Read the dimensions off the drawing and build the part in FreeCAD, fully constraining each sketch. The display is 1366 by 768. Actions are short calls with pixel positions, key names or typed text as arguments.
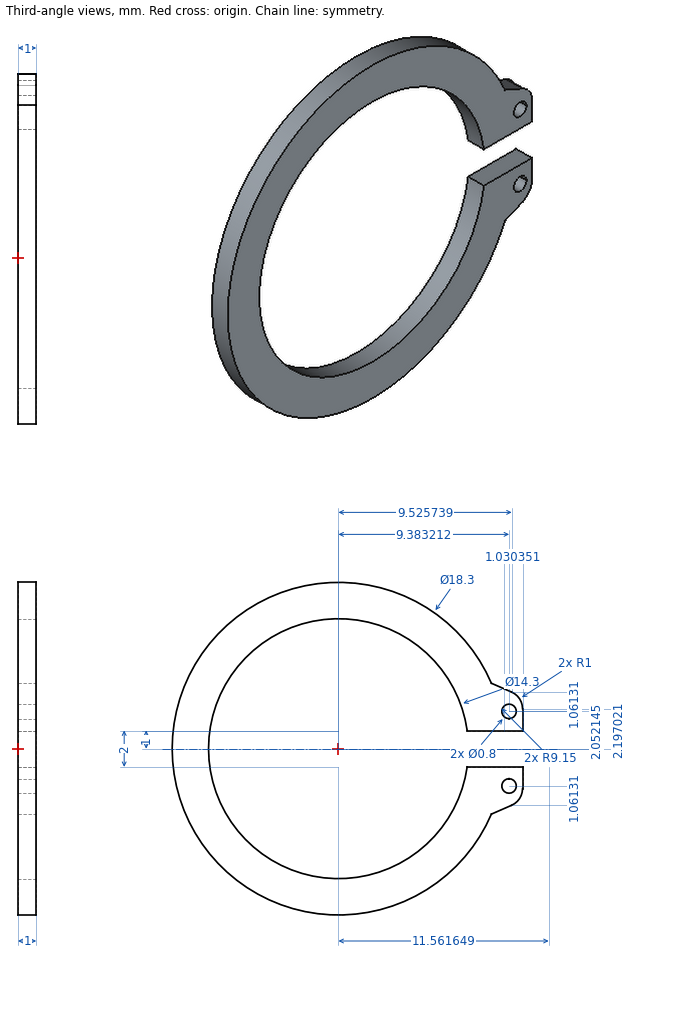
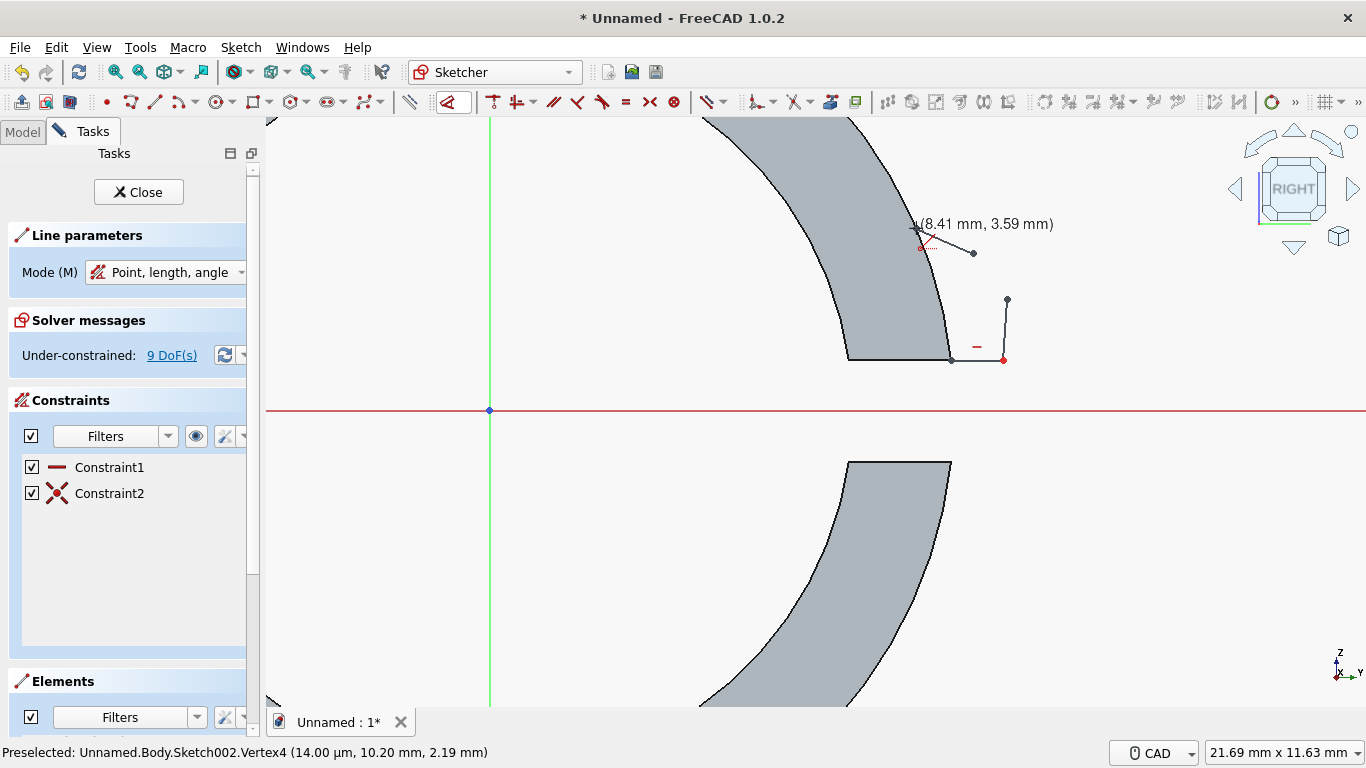
key(g)
key(3)
key(a)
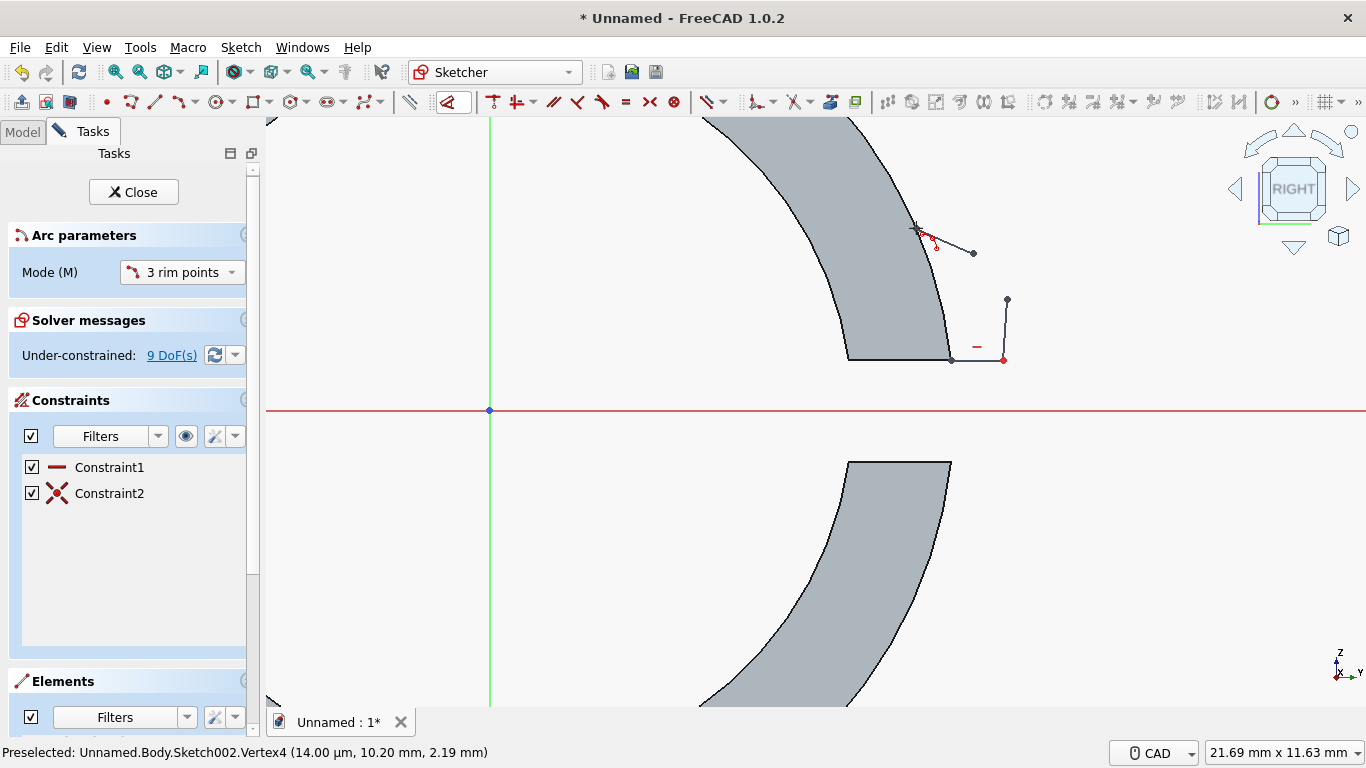
click(1007, 300)
click(973, 254)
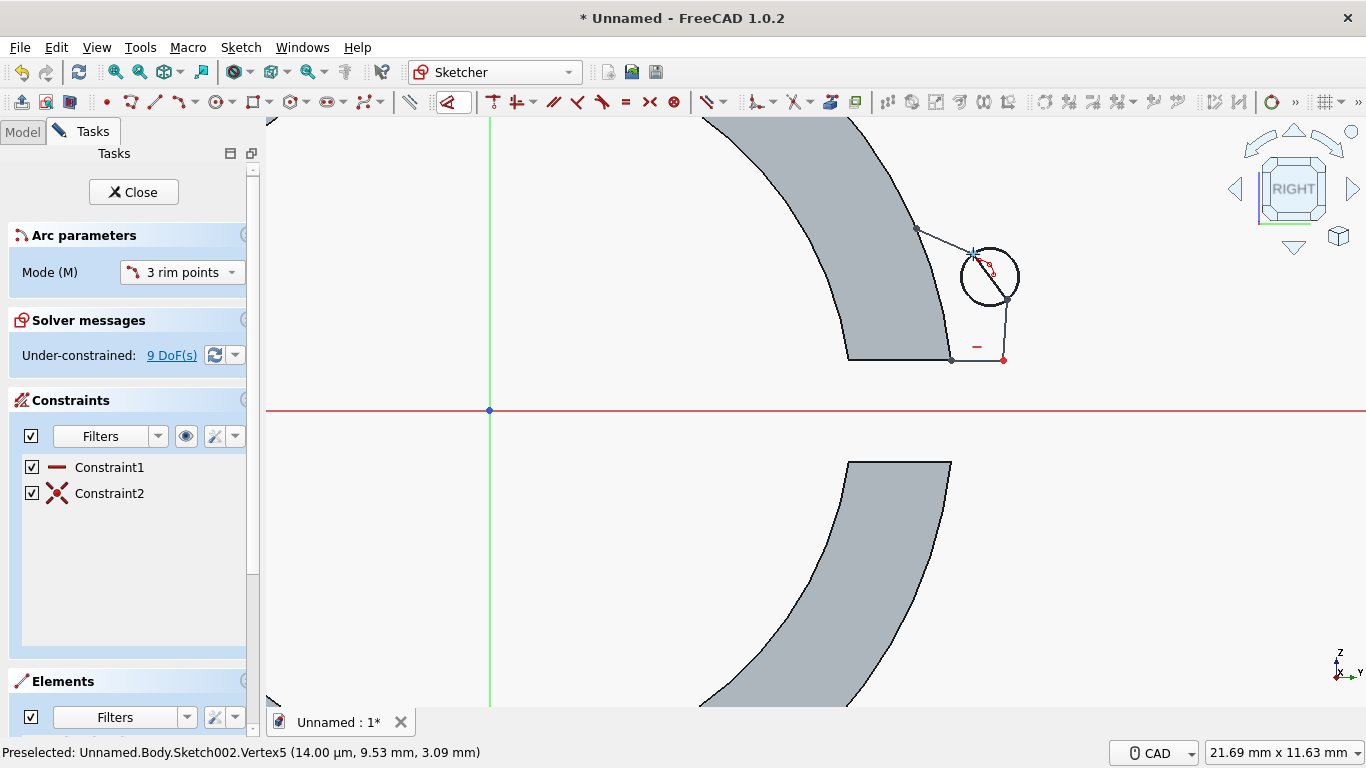
scroll(995, 272, up, 4)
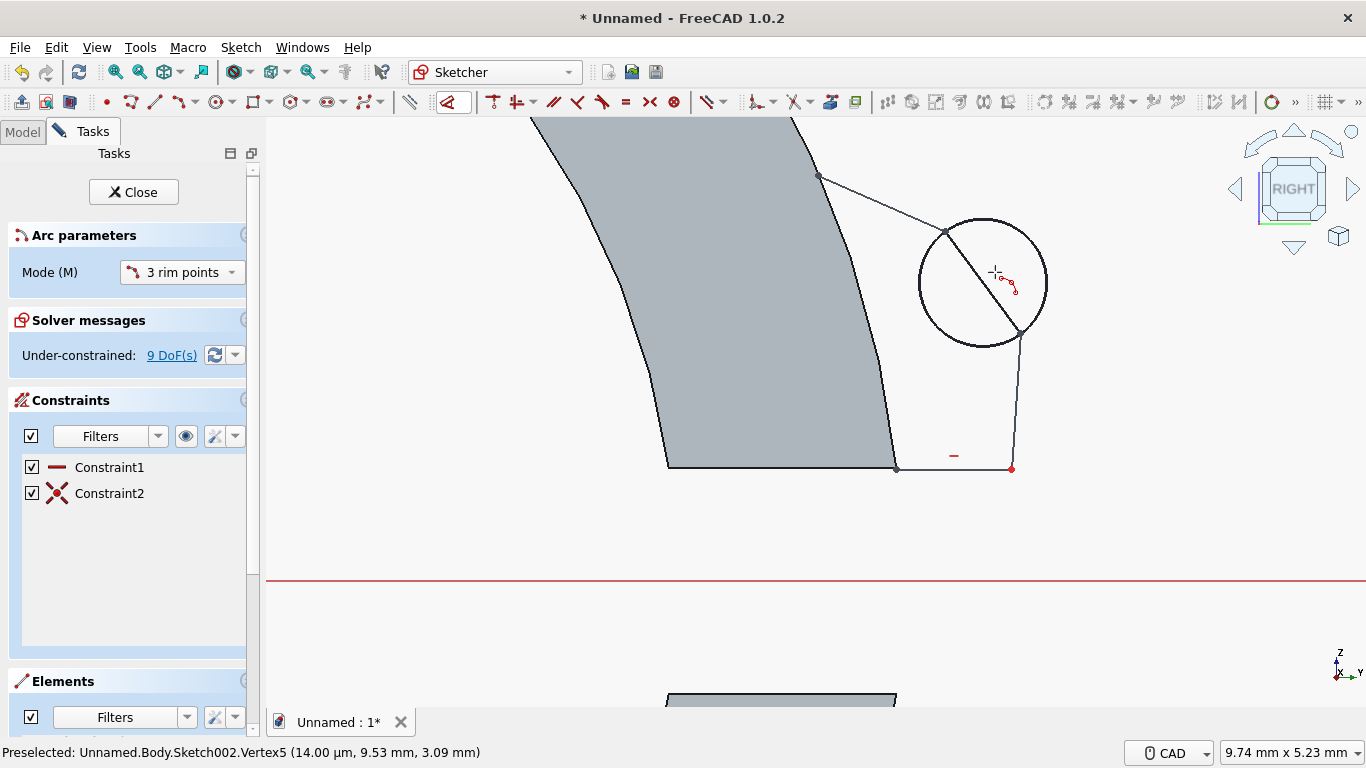
click(994, 271)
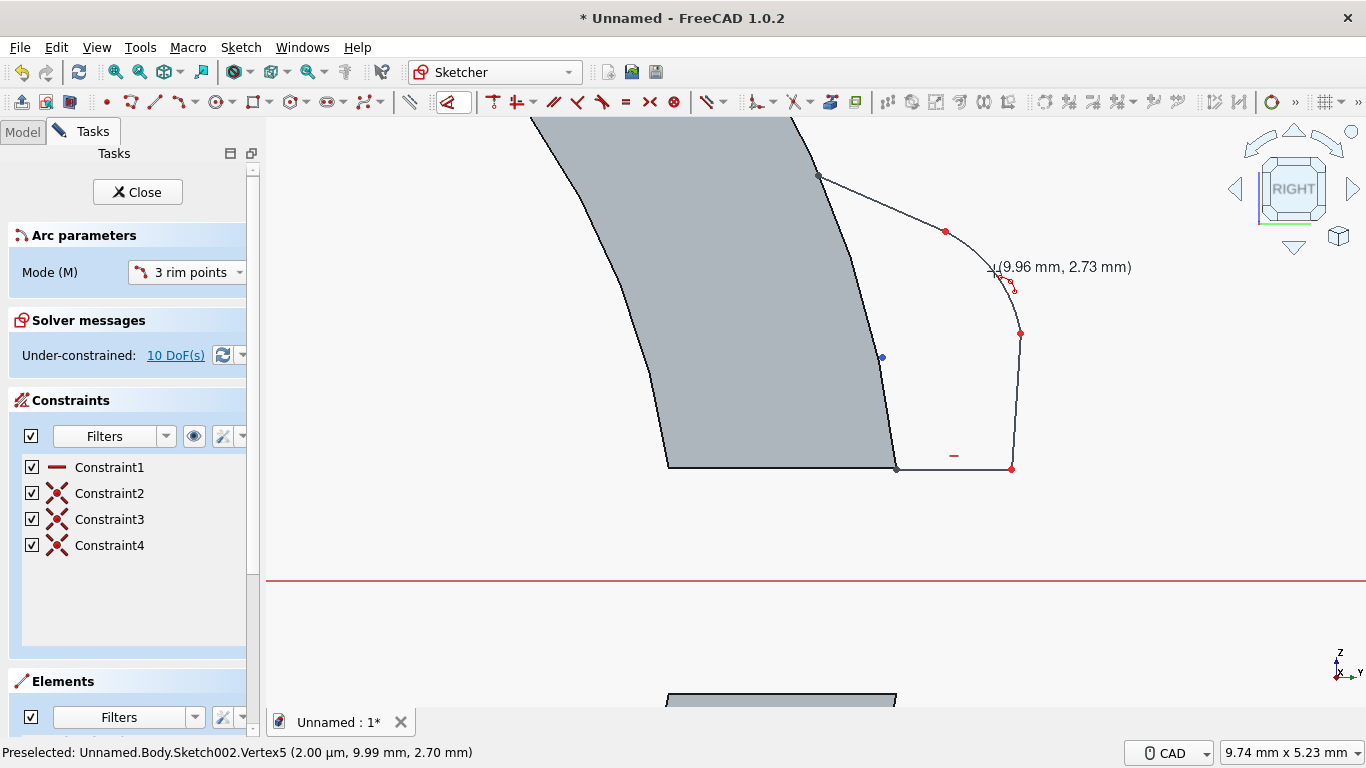
click(818, 176)
click(896, 470)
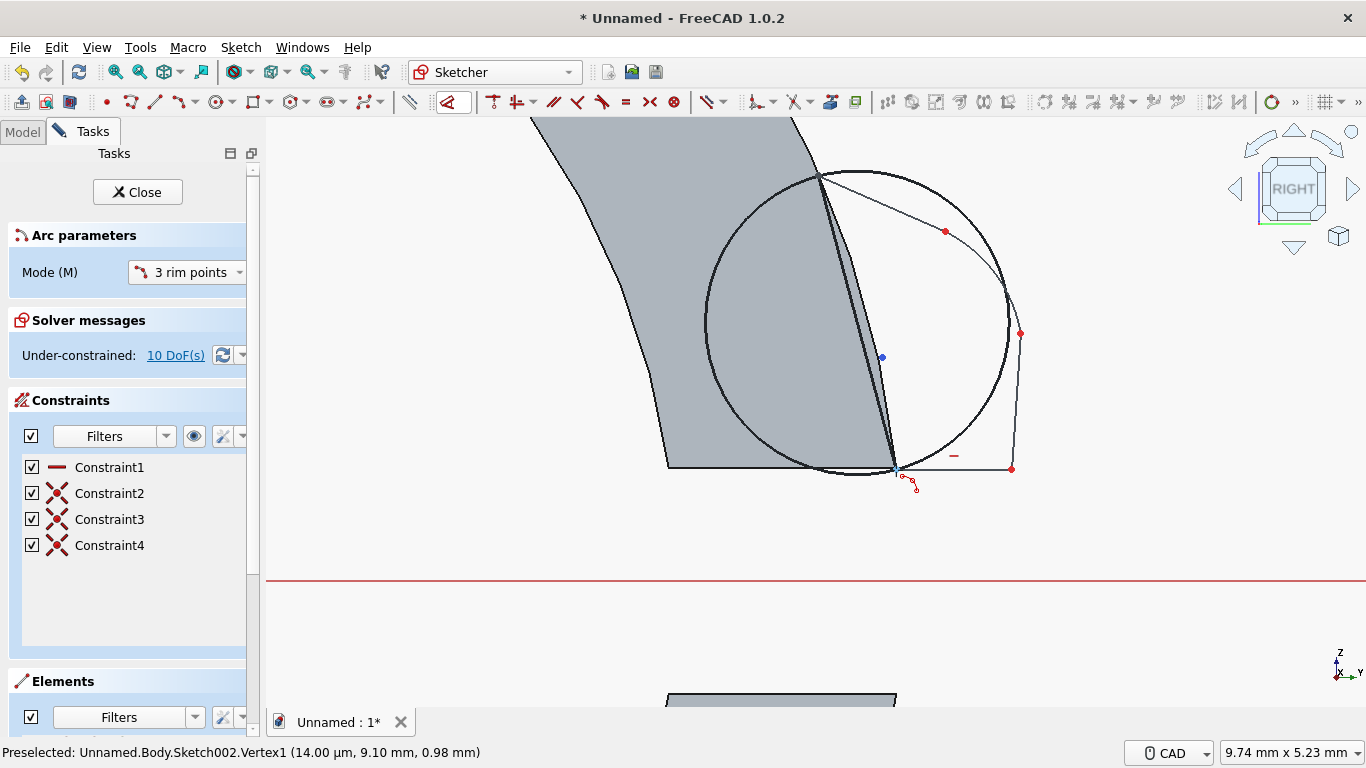
scroll(869, 318, up, 2)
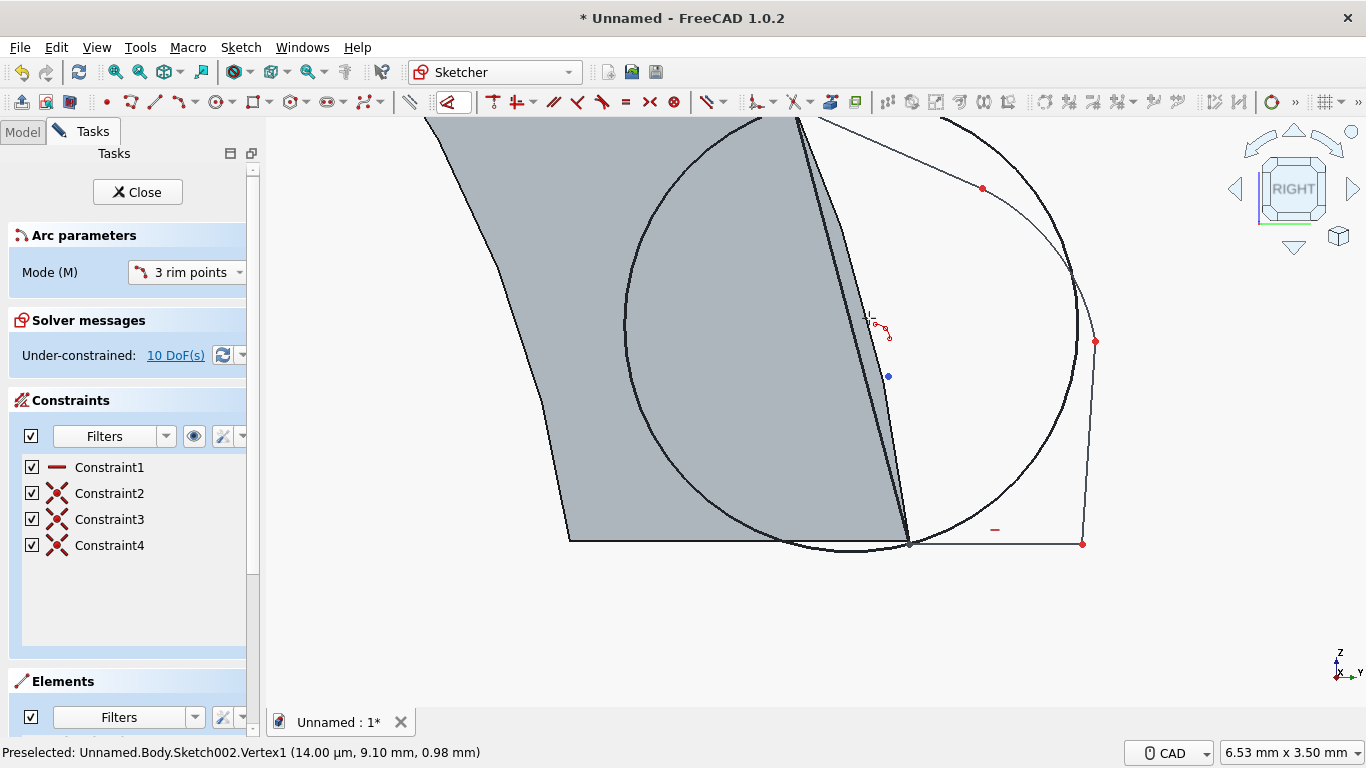
click(868, 318)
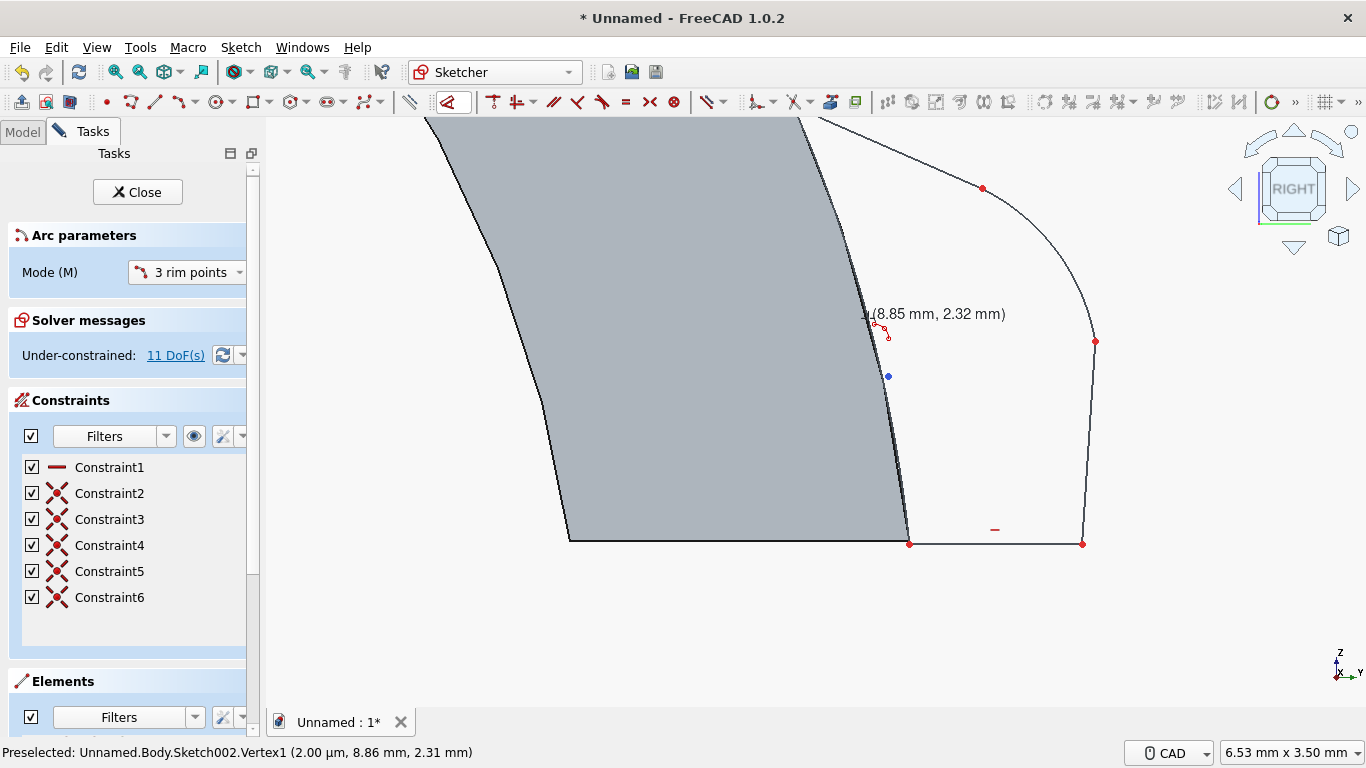
key(g)
key(l)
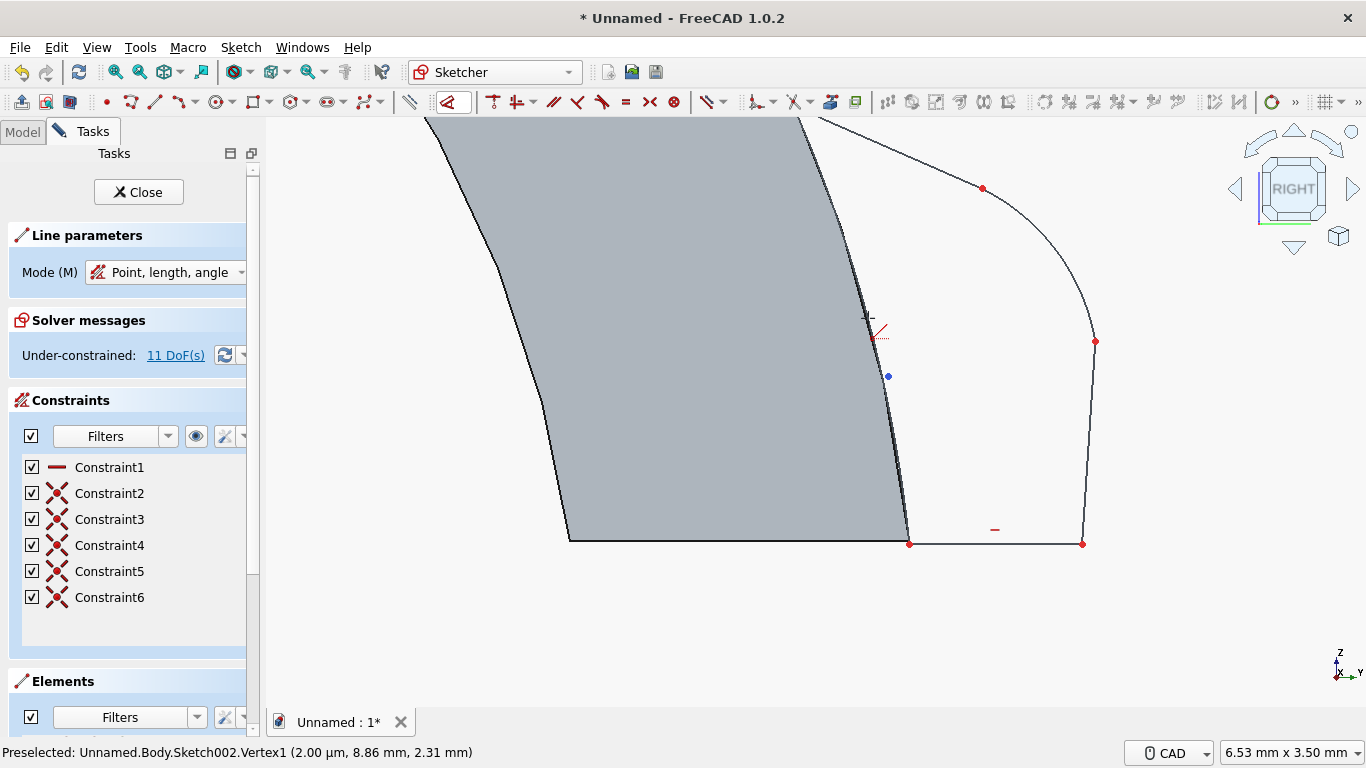
scroll(970, 284, down, 6)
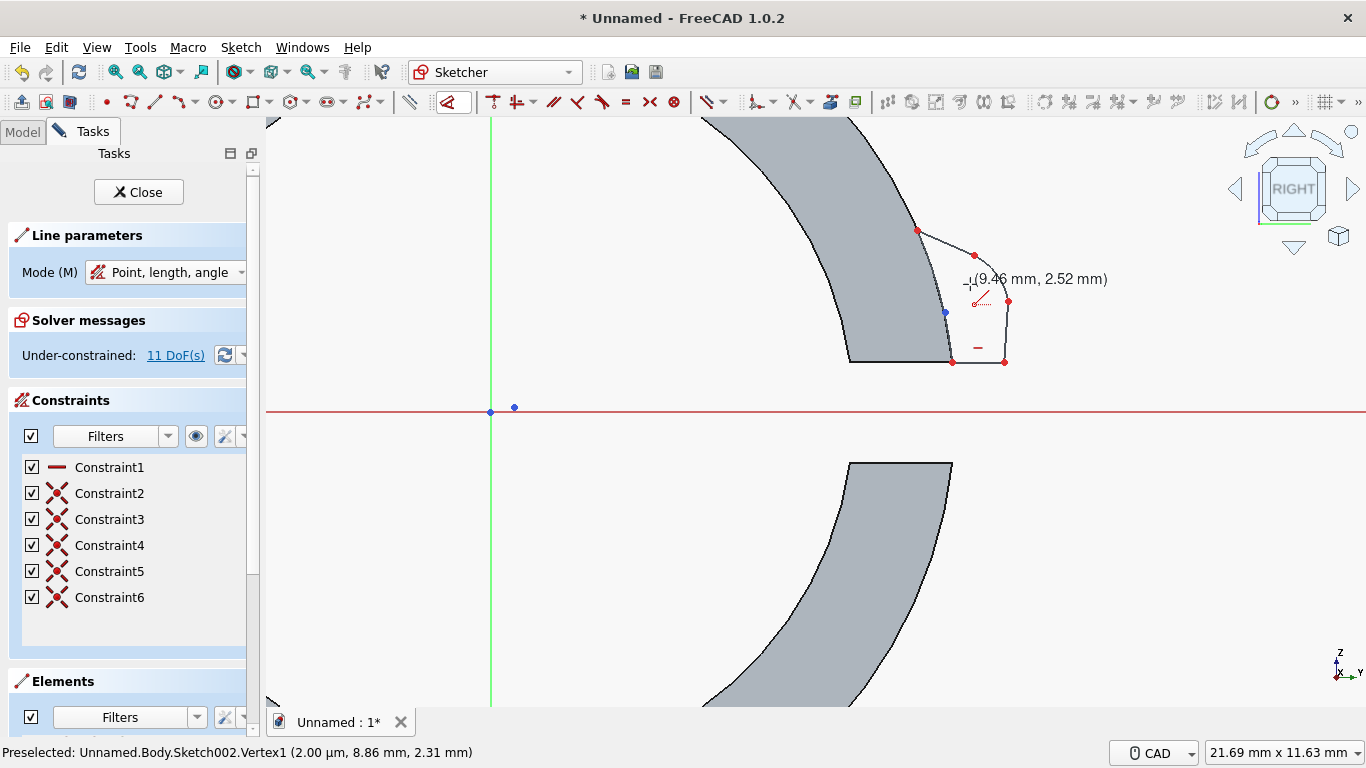
click(918, 595)
click(974, 570)